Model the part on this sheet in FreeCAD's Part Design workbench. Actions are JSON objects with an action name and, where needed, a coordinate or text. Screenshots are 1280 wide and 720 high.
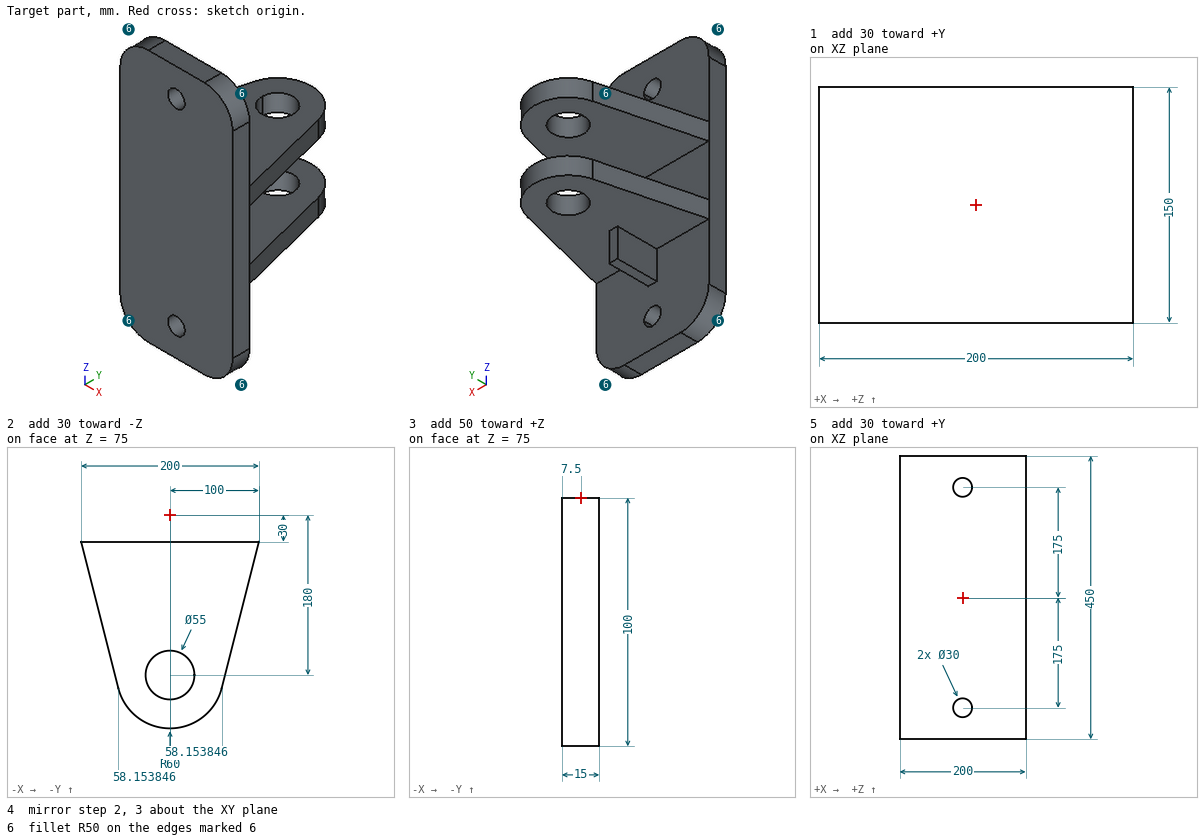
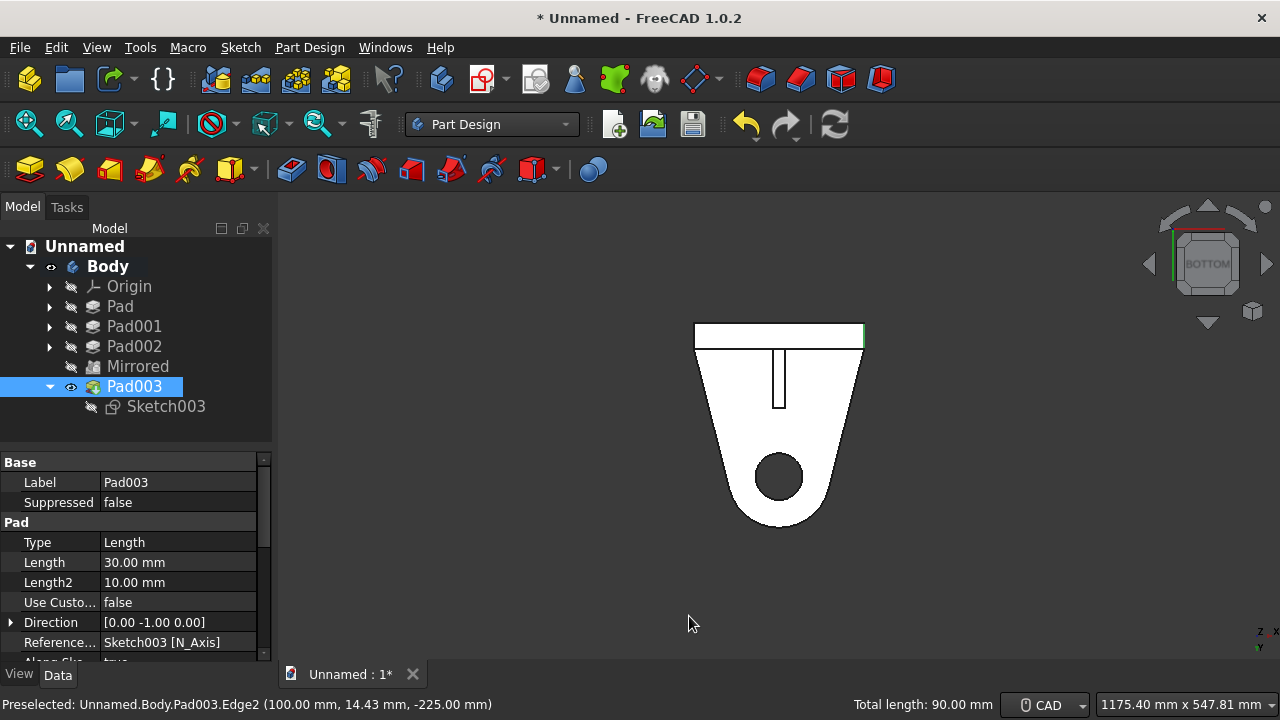
{"action": "left_click", "coordinate": [694, 335], "text": "ctrl"}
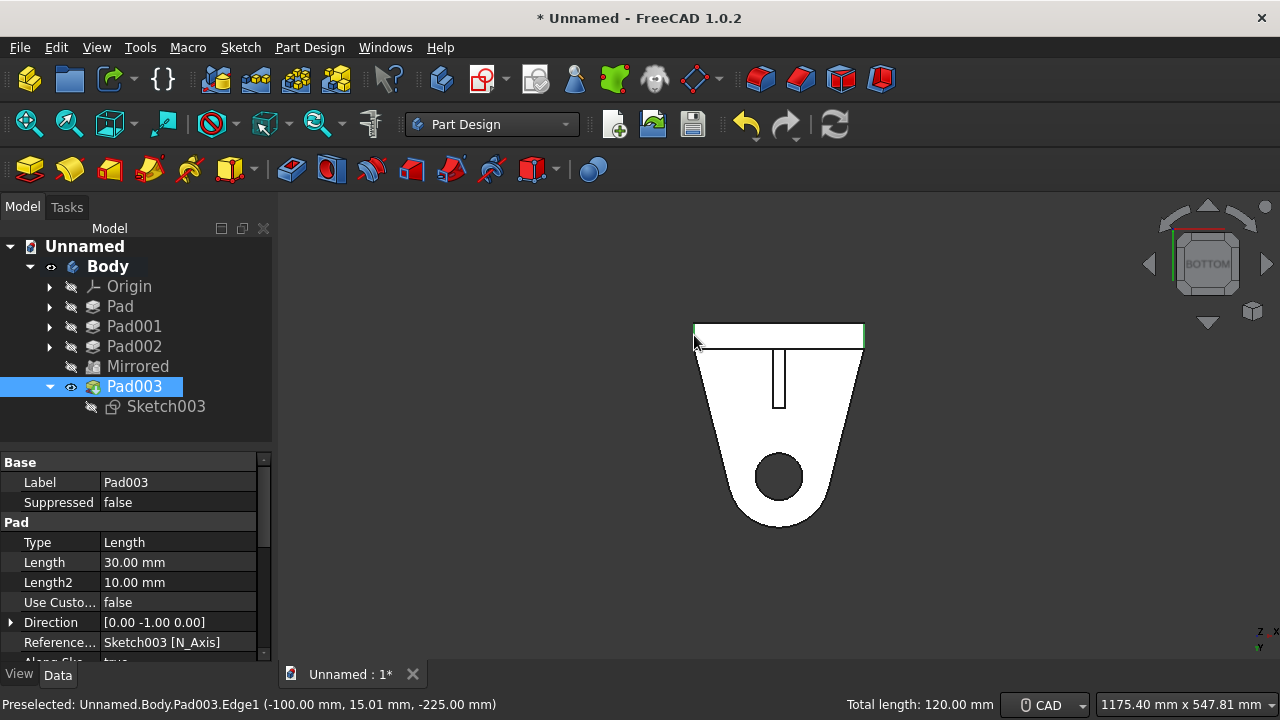
{"action": "left_click", "coordinate": [762, 80]}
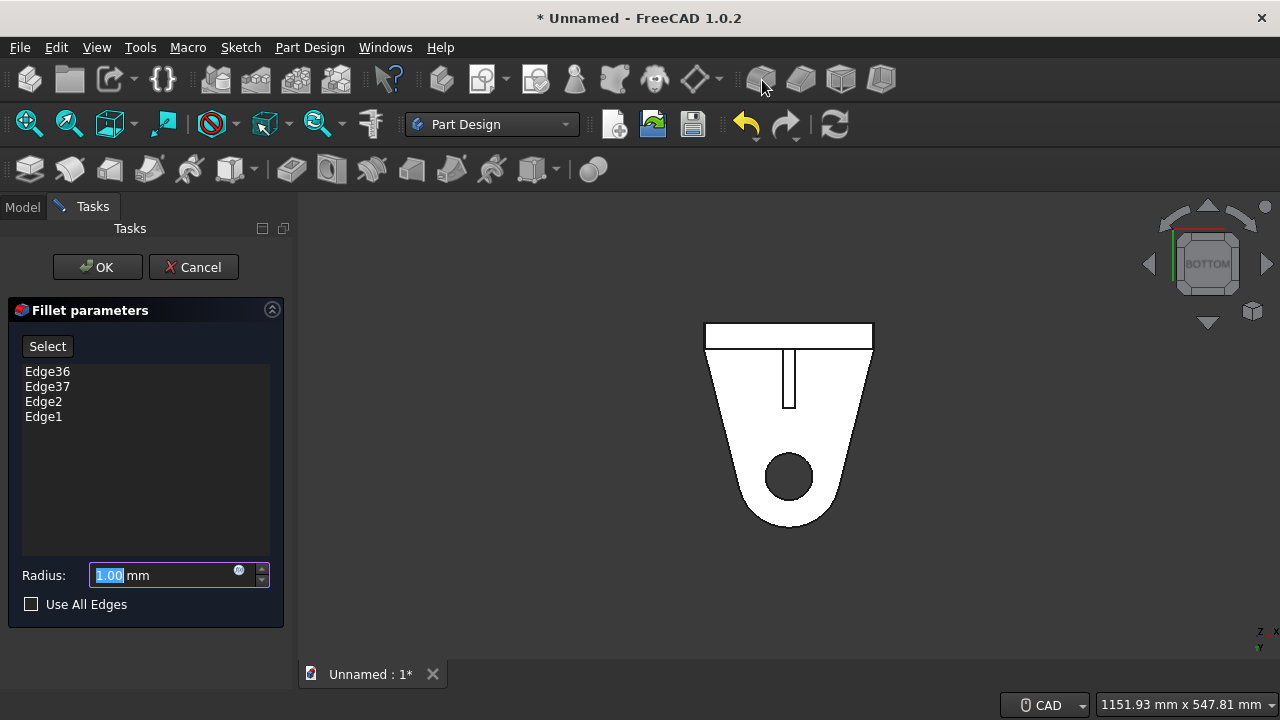
{"action": "type", "text": "50"}
{"action": "key", "text": "Tab"}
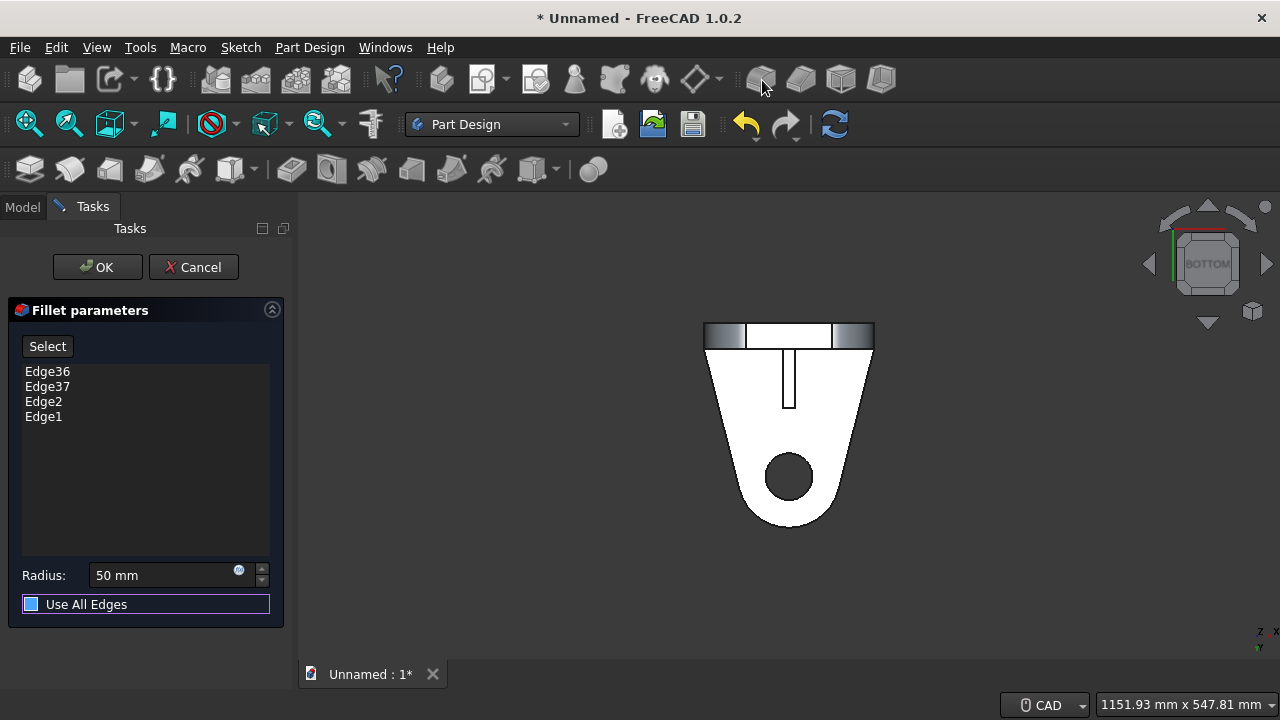
{"action": "left_click", "coordinate": [98, 267]}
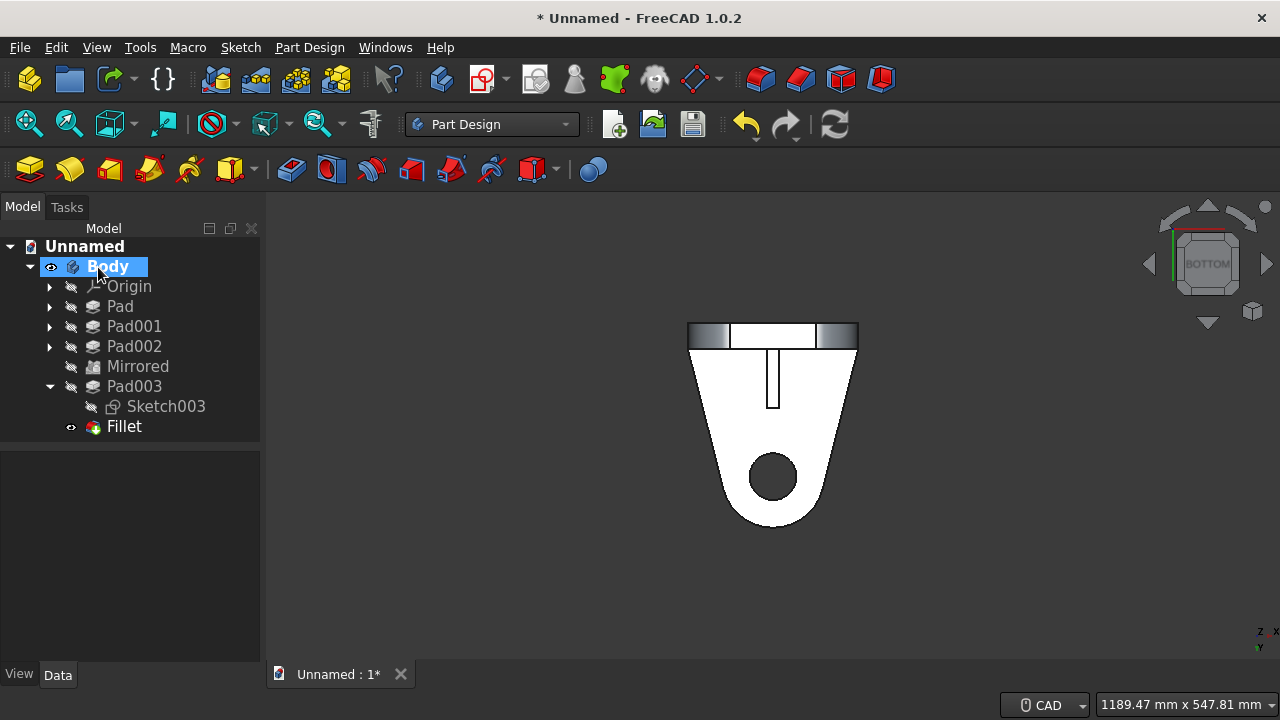
{"action": "key", "text": "0"}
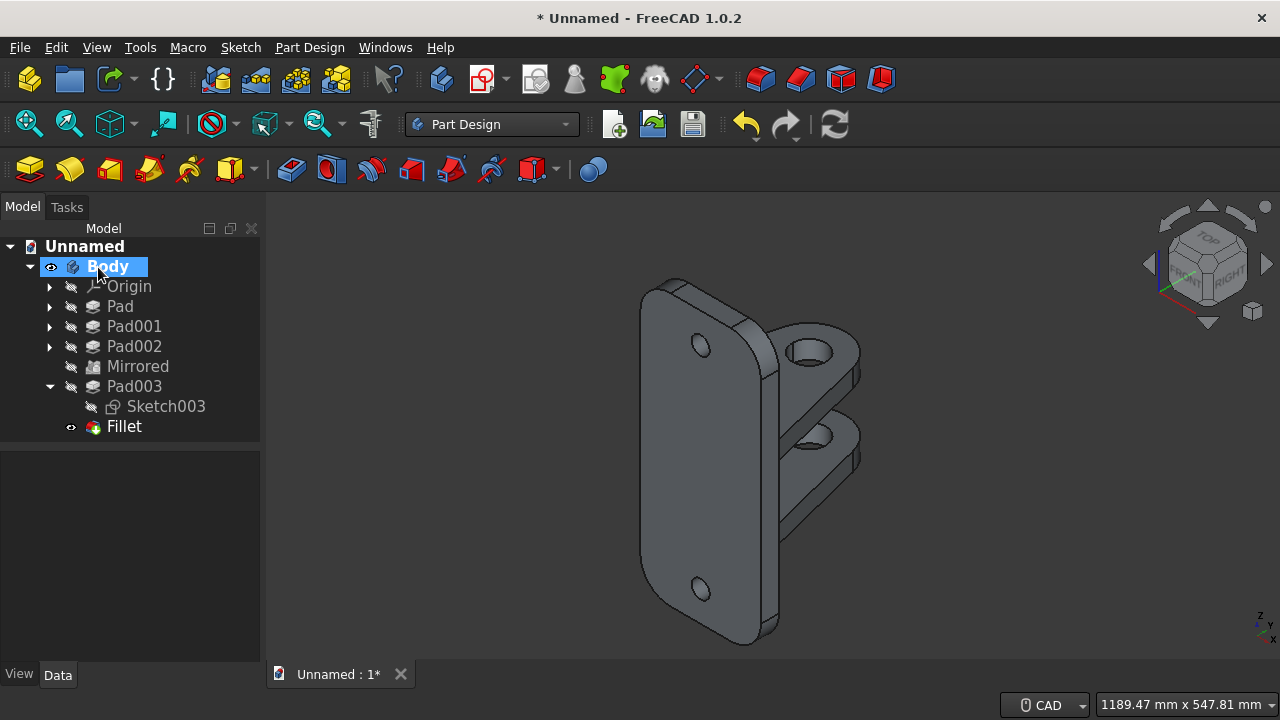
{"action": "key", "text": "v f"}